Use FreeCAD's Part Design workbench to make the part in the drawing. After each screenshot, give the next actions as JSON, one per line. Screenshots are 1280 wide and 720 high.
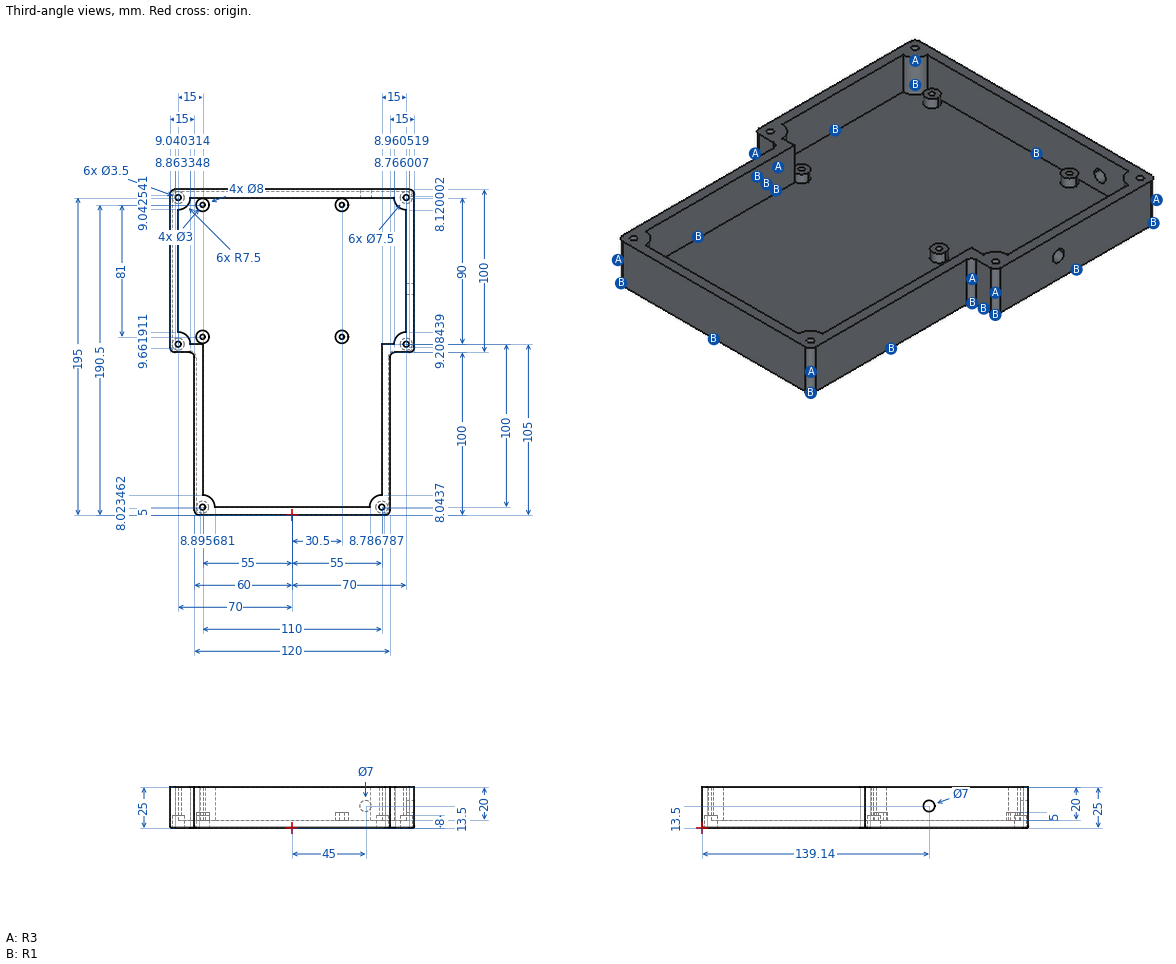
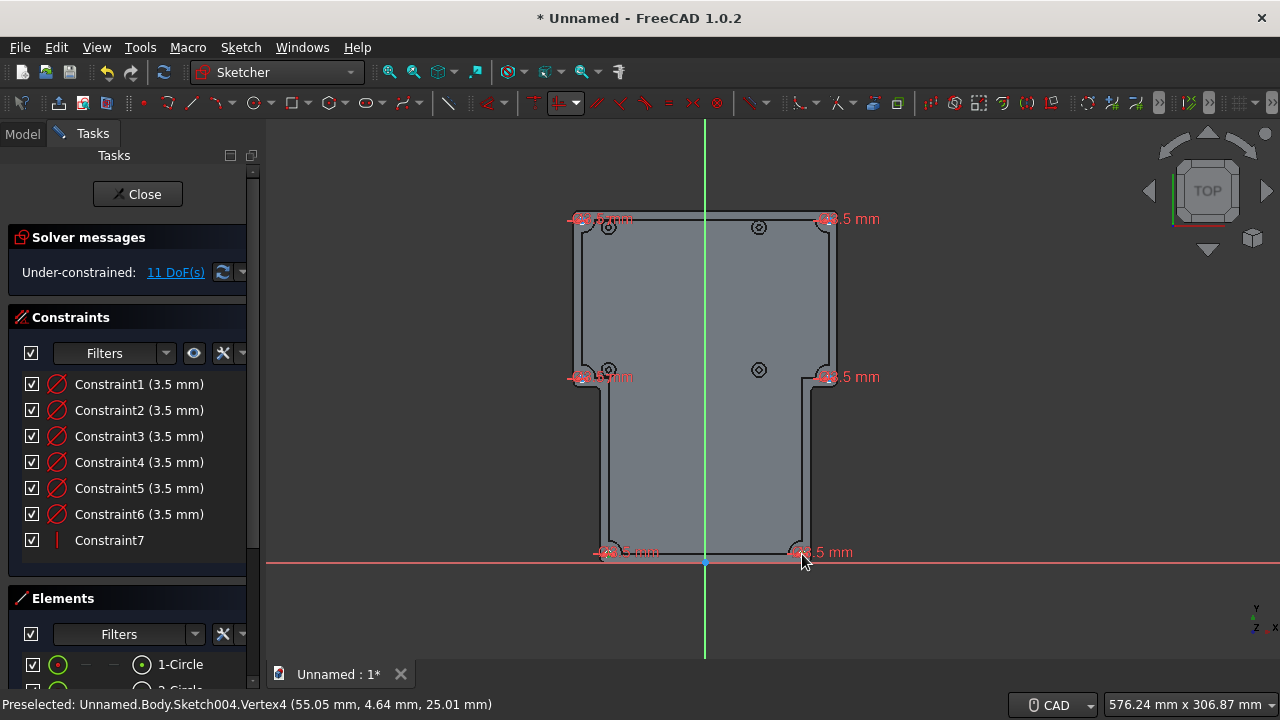
{"action": "key", "text": "h"}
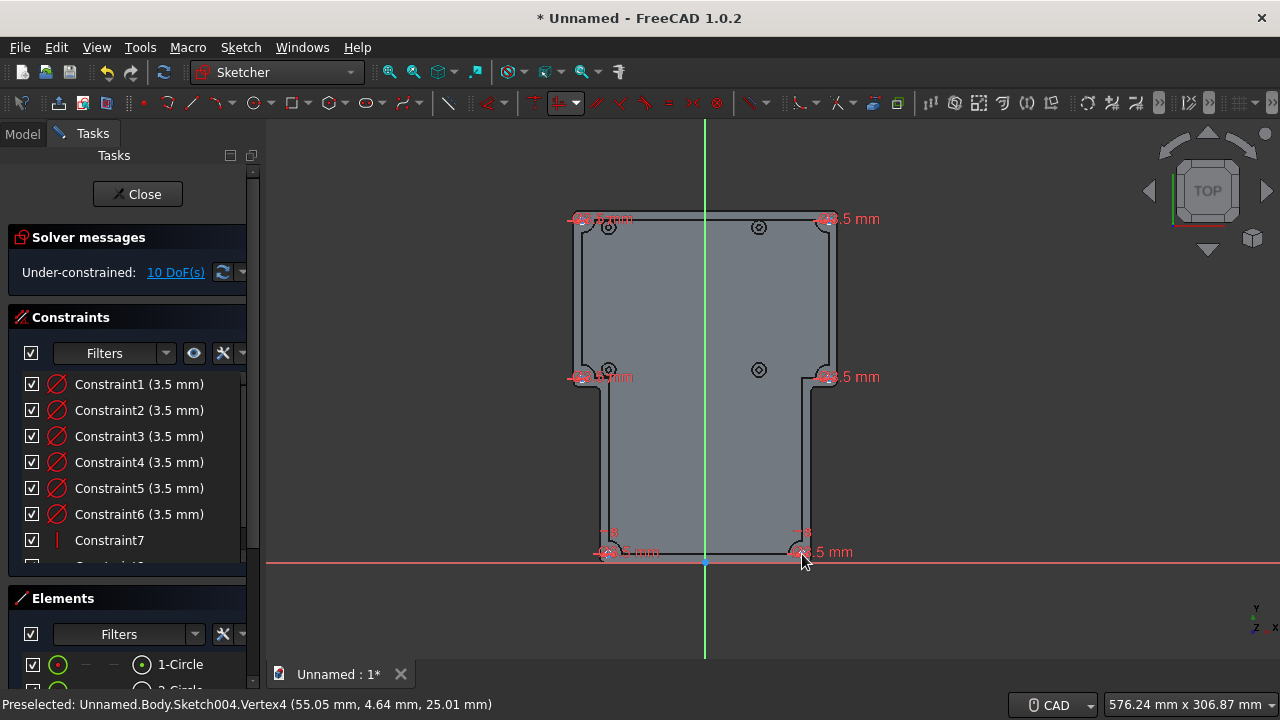
{"action": "left_click", "coordinate": [582, 379]}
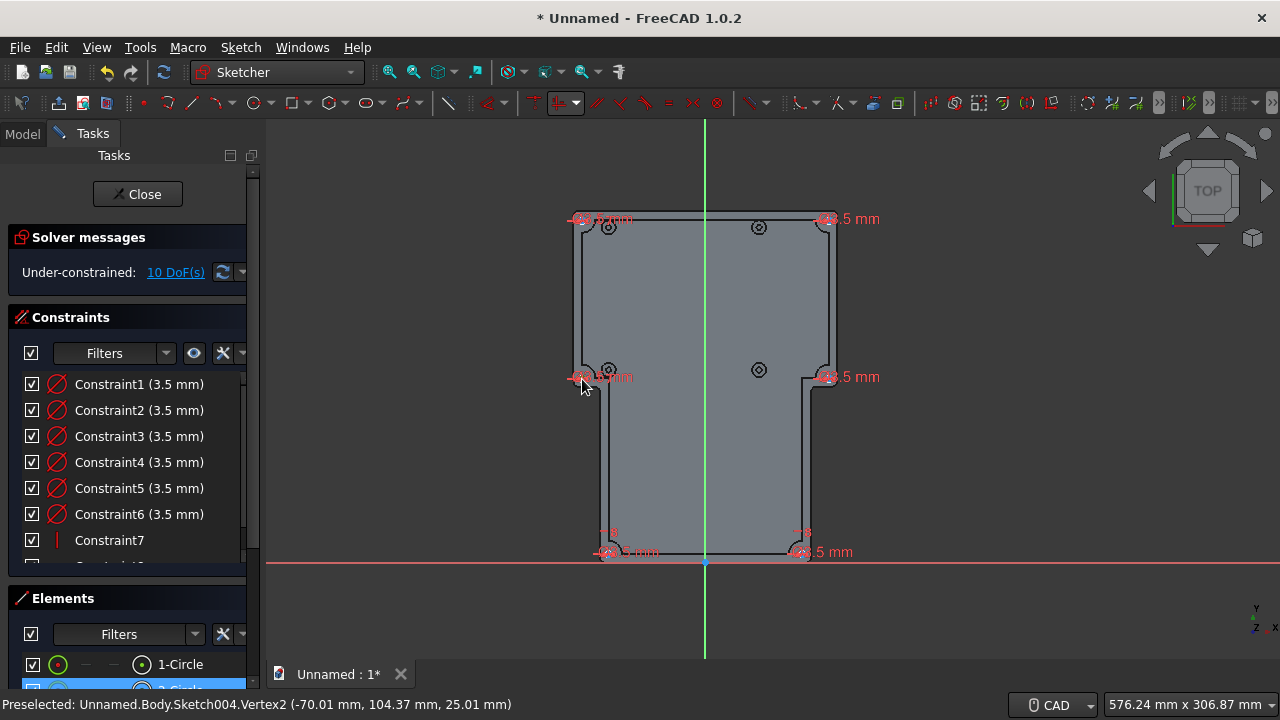
{"action": "left_click", "coordinate": [829, 379]}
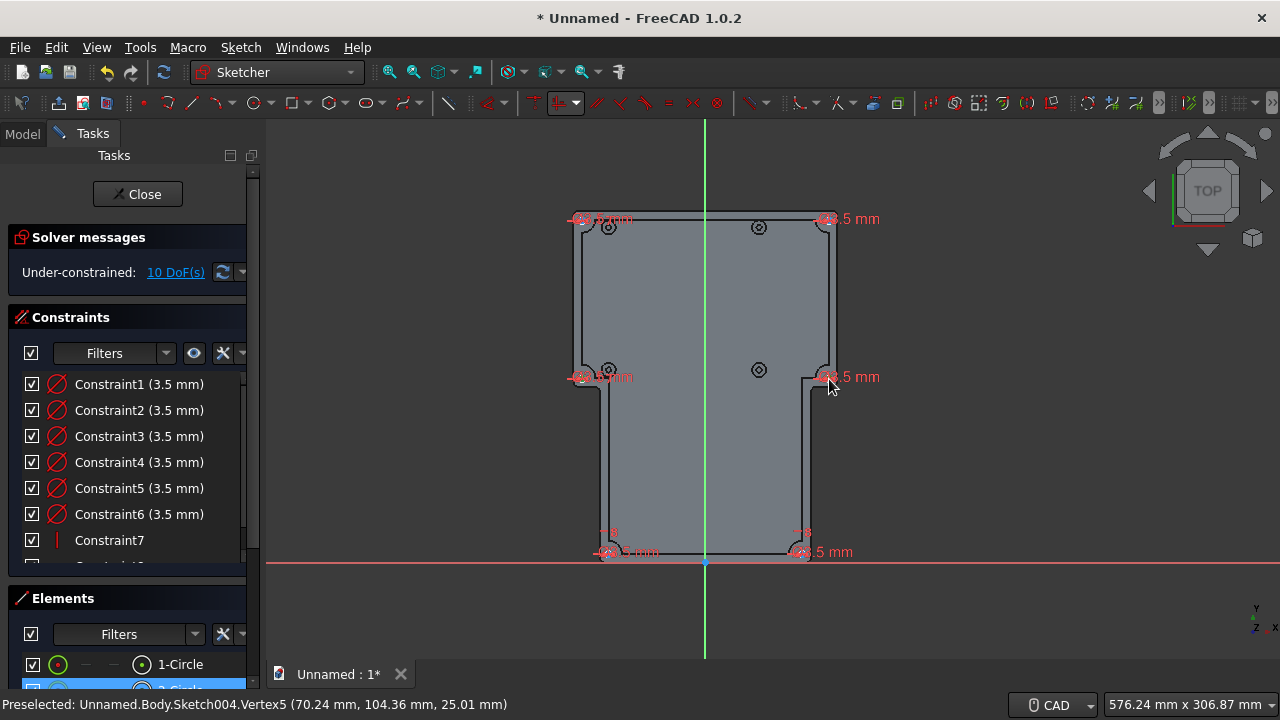
{"action": "key", "text": "h"}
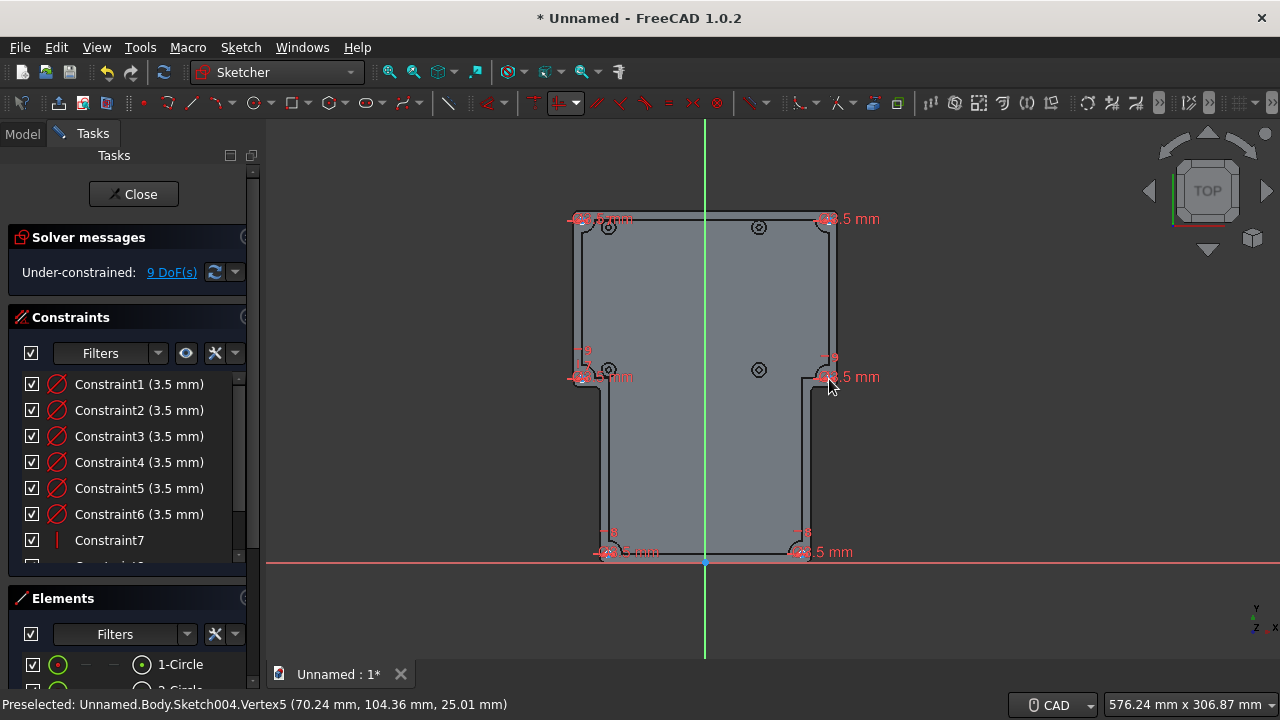
{"action": "left_click", "coordinate": [829, 379]}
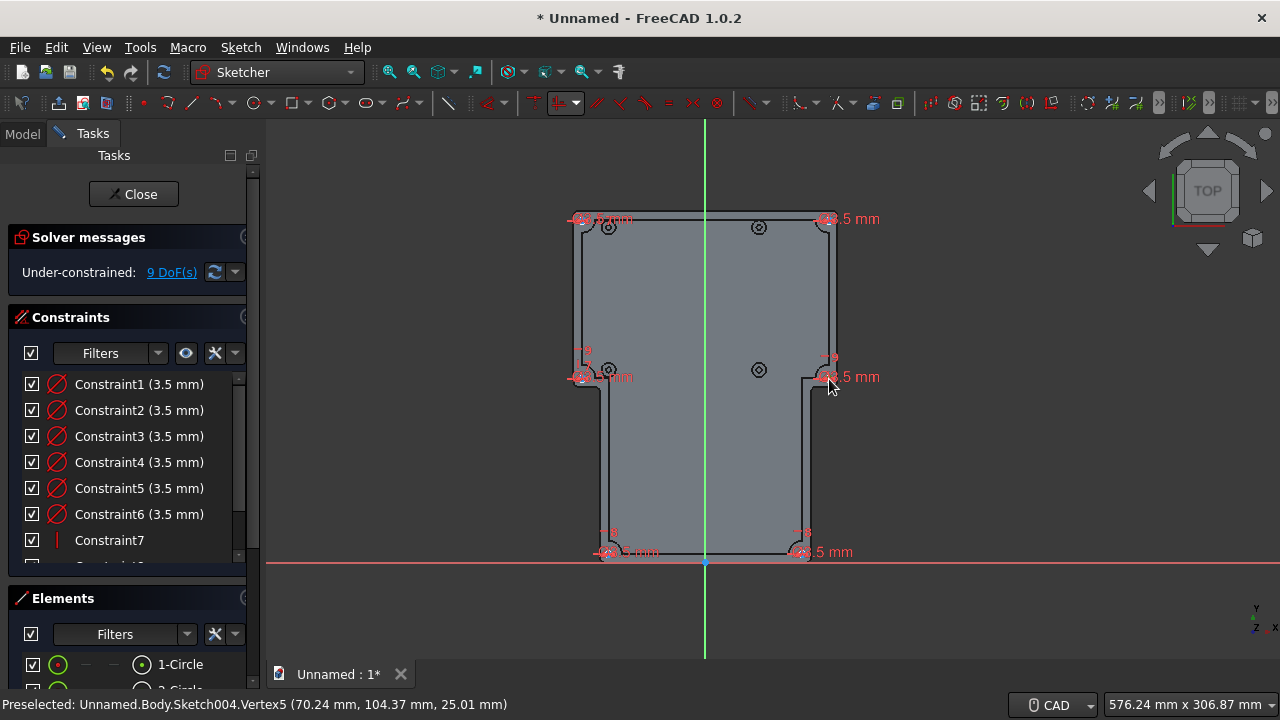
{"action": "left_click", "coordinate": [829, 221]}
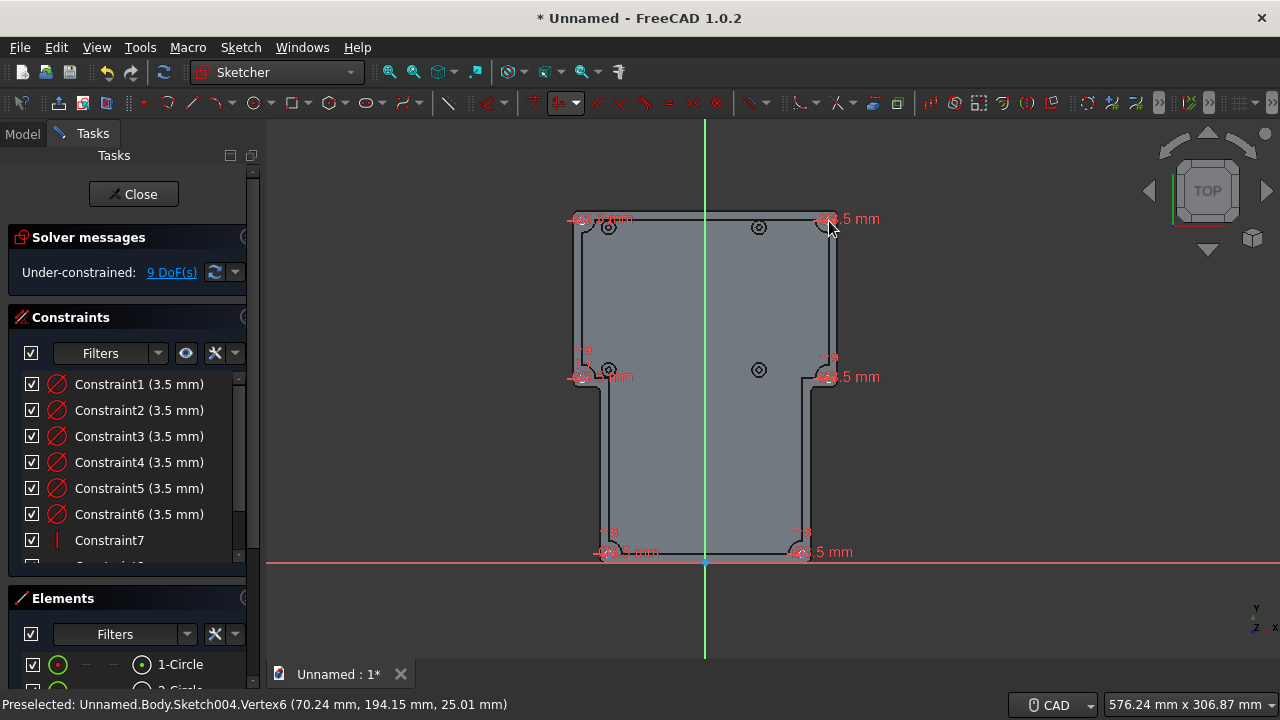
{"action": "left_click", "coordinate": [578, 104]}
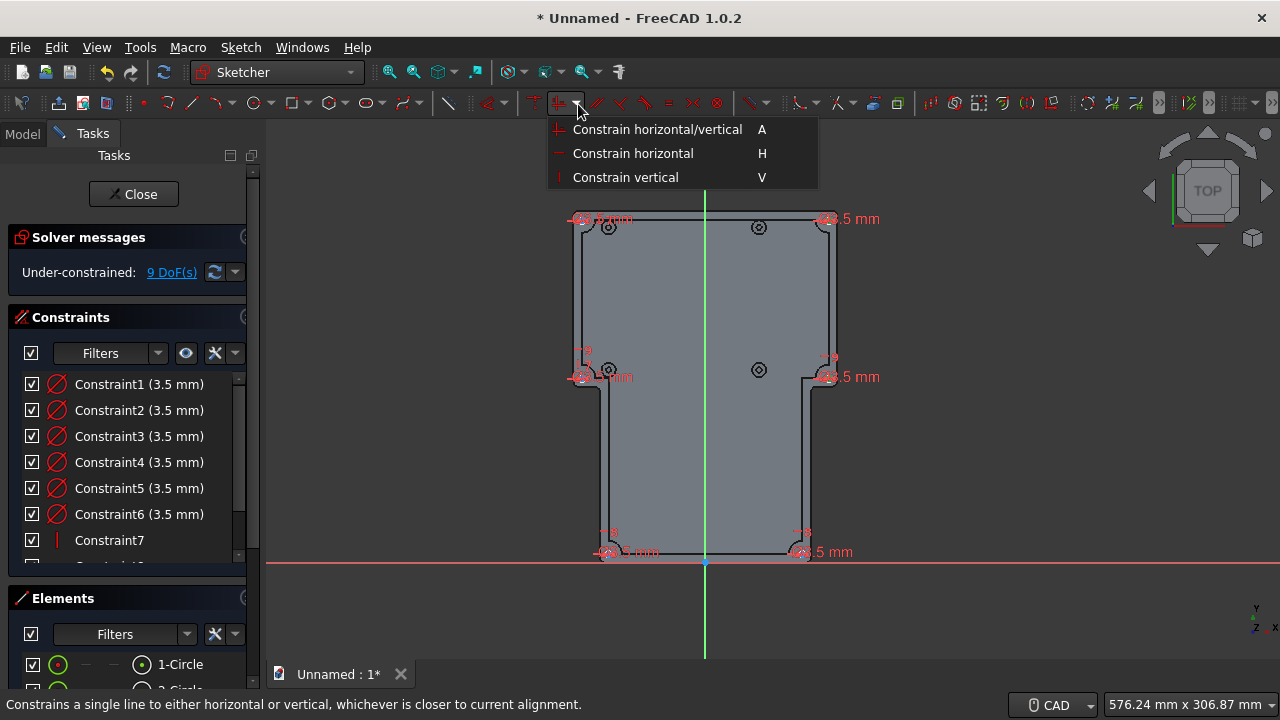
{"action": "left_click", "coordinate": [683, 177]}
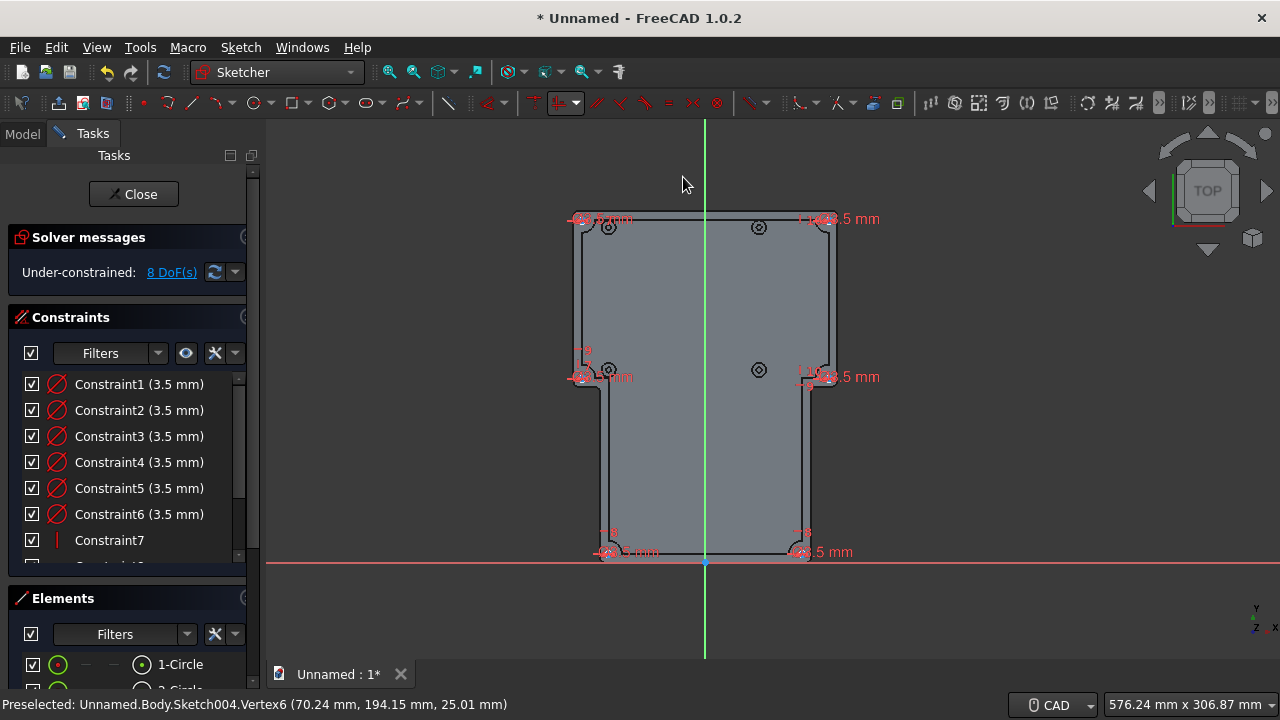
{"action": "left_click", "coordinate": [582, 221]}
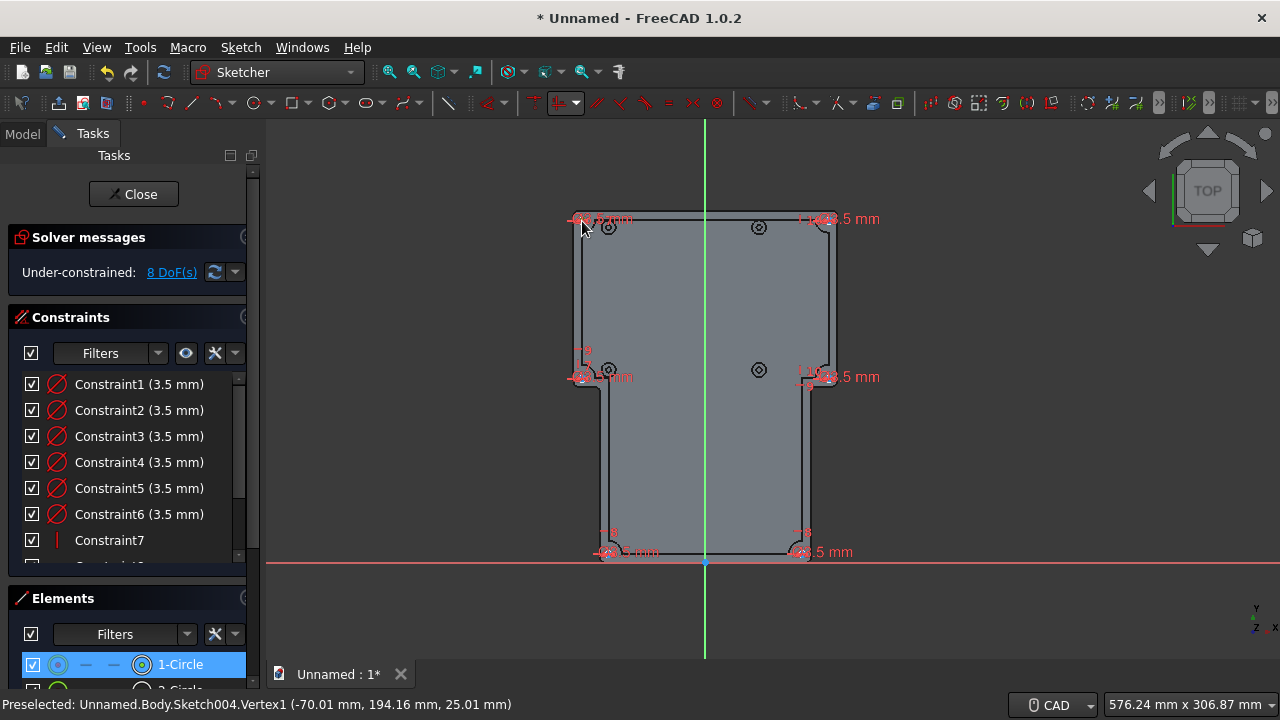
{"action": "left_click", "coordinate": [829, 221]}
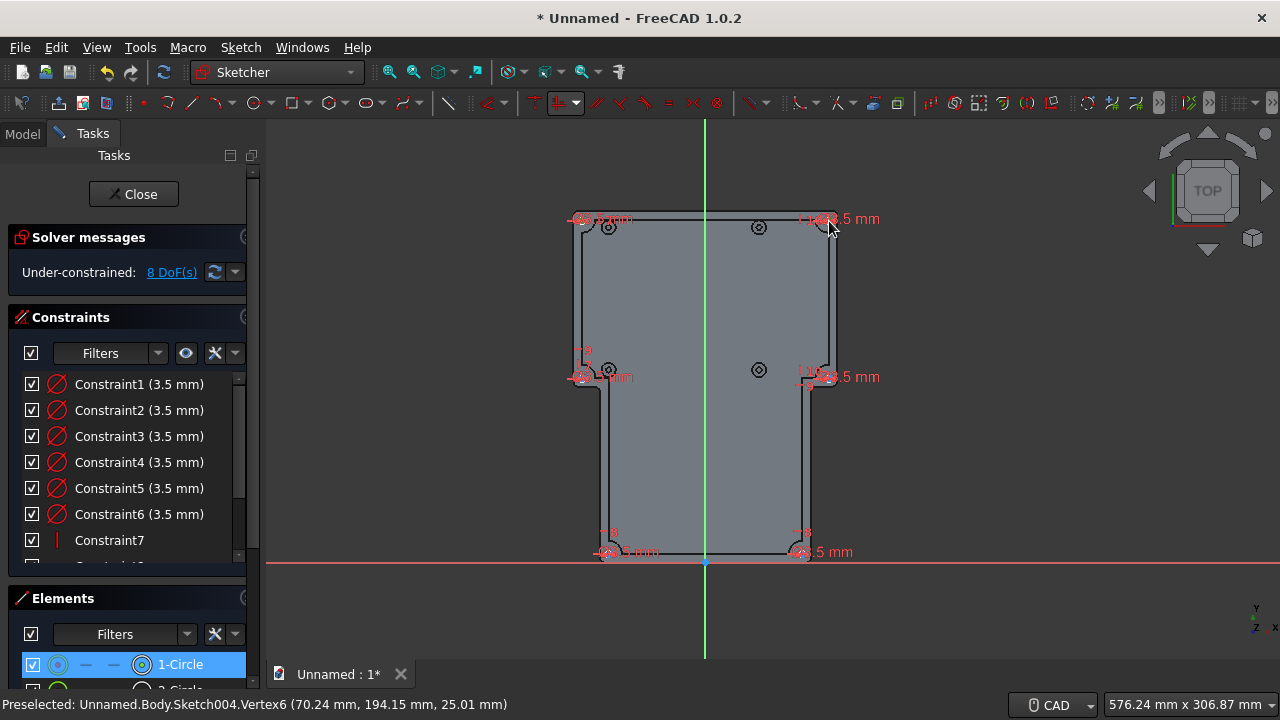
{"action": "key", "text": "h"}